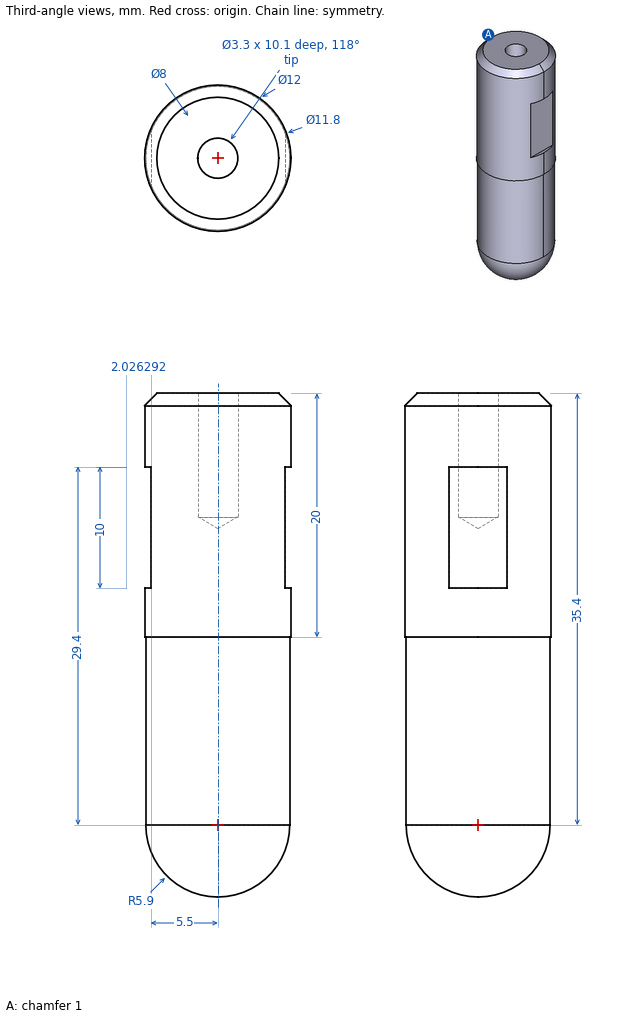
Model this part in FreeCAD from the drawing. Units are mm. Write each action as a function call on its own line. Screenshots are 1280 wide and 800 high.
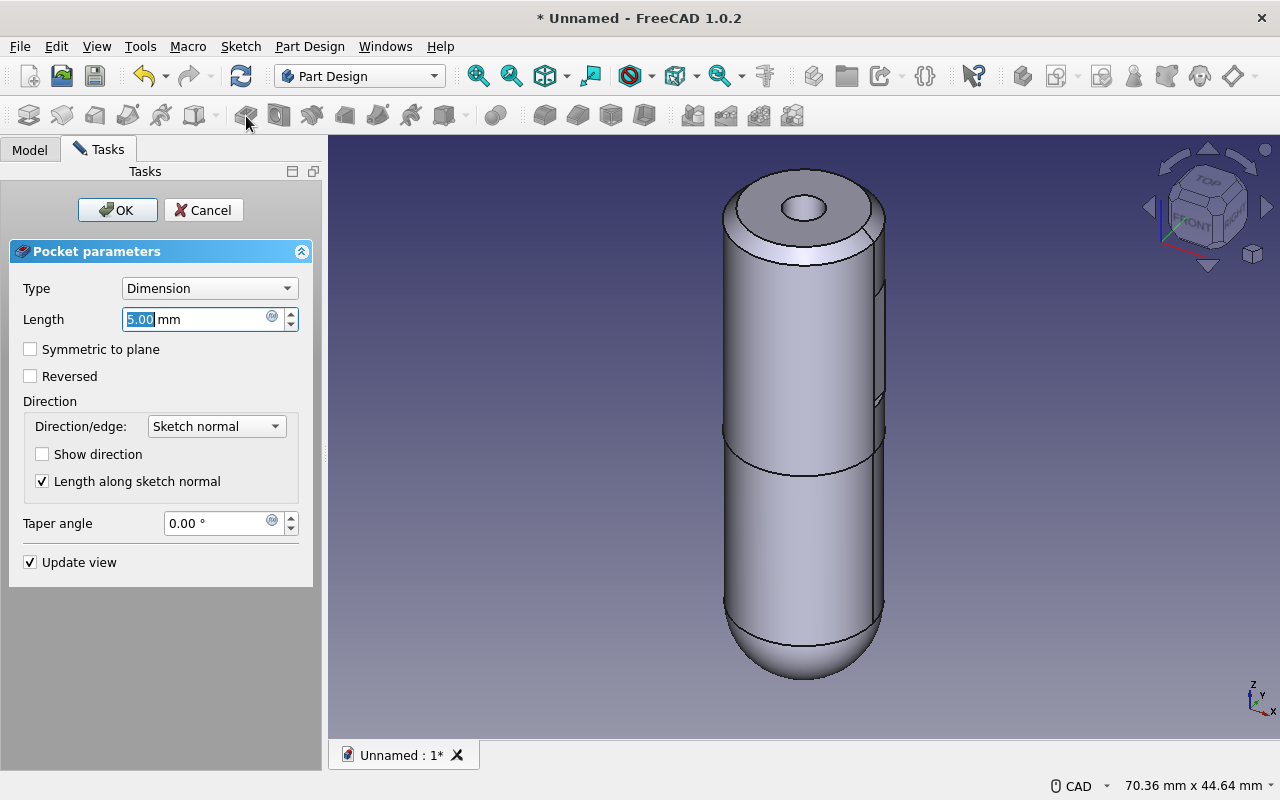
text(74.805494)
key(Tab)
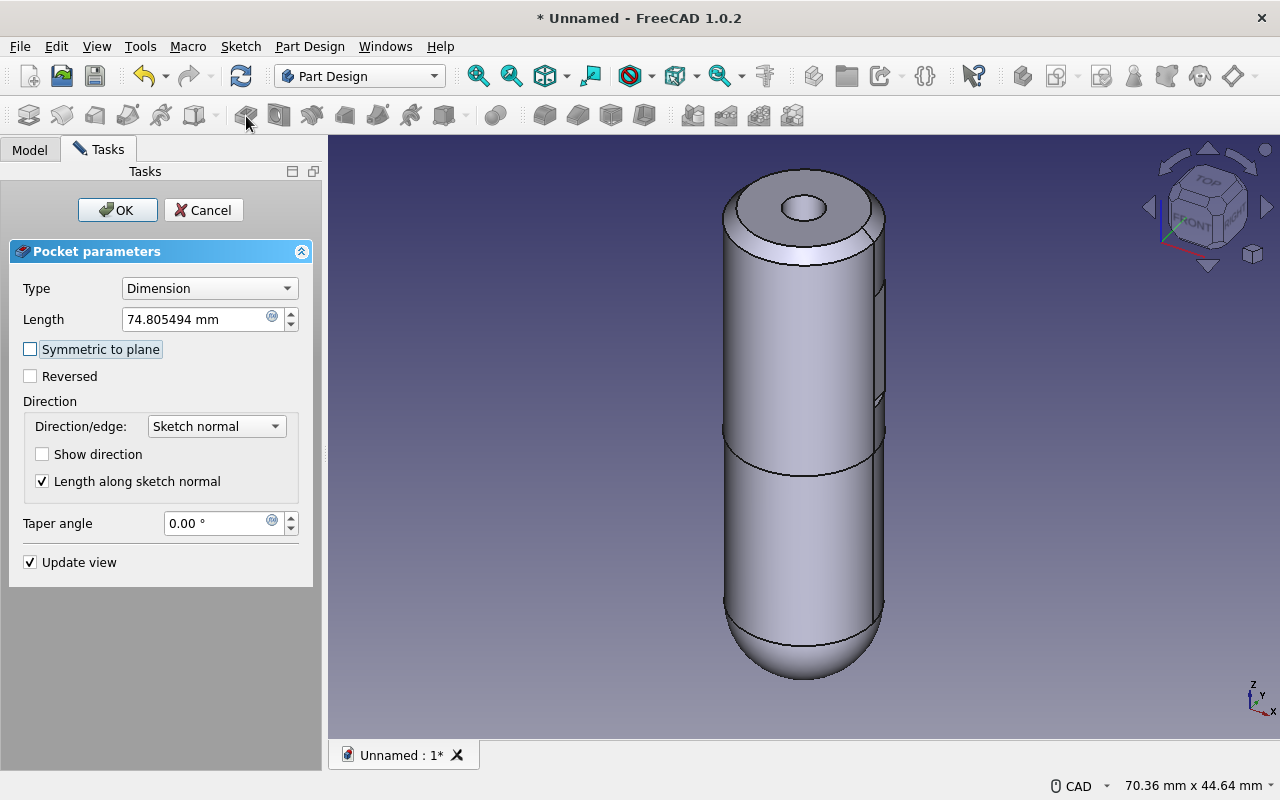
click(31, 349)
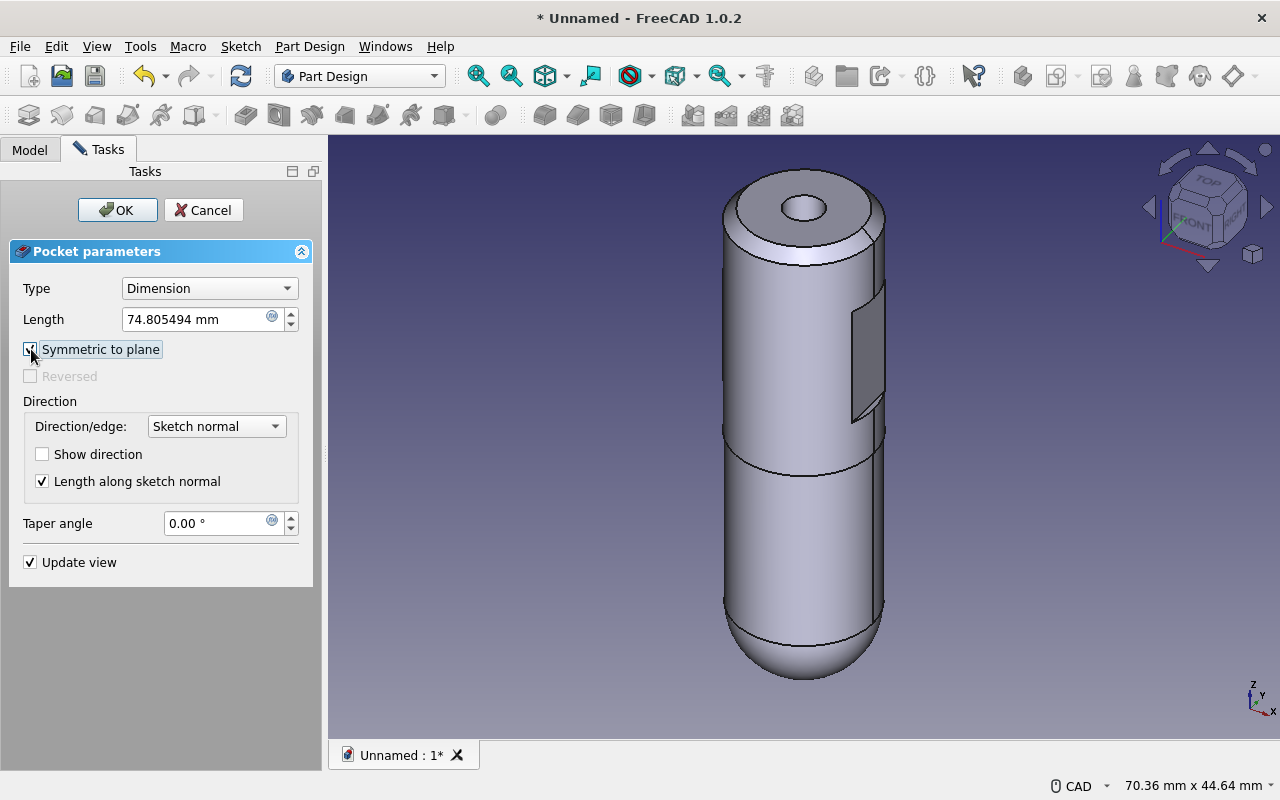
click(118, 210)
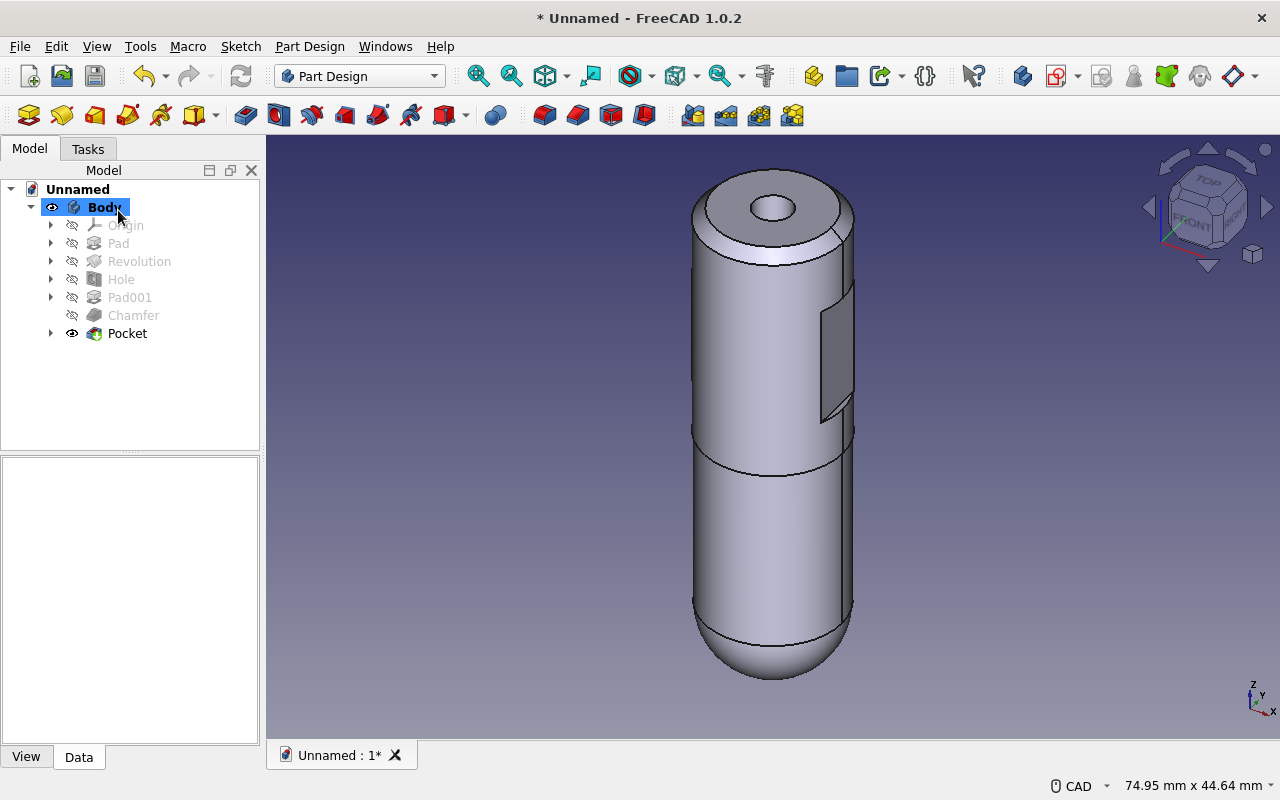
key(0)